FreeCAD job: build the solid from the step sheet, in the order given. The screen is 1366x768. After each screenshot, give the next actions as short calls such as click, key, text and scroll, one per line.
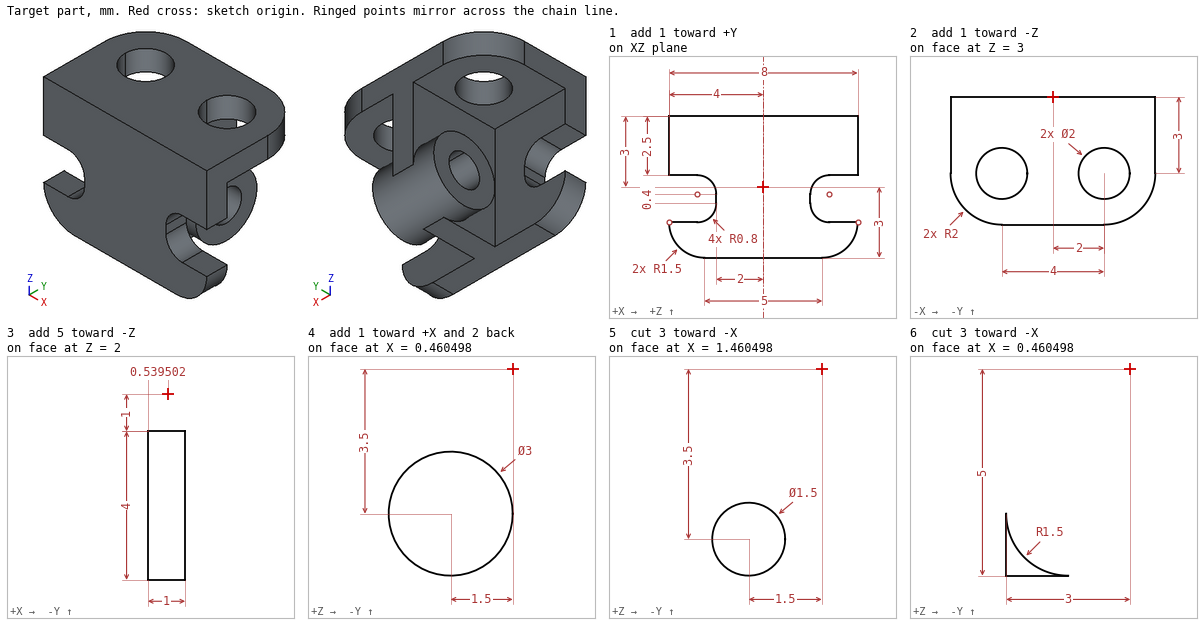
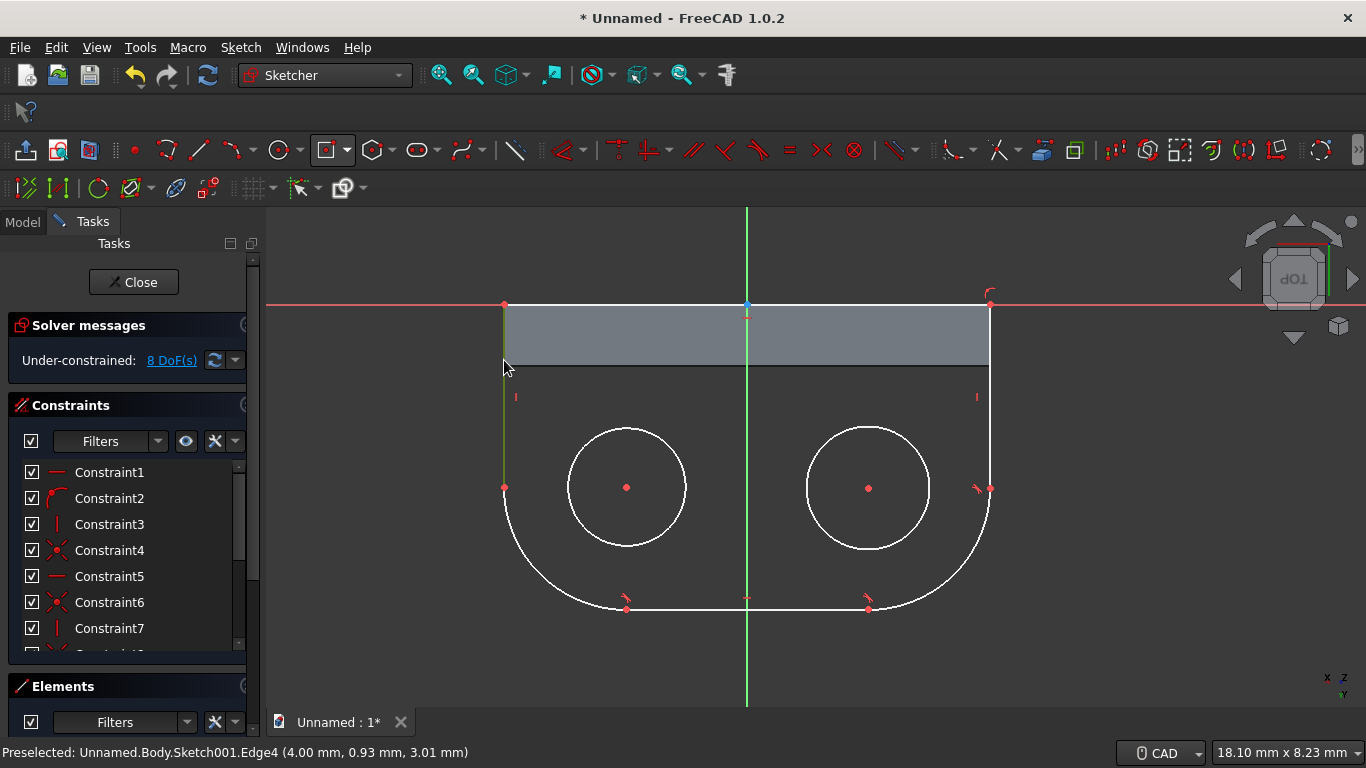
click(518, 543)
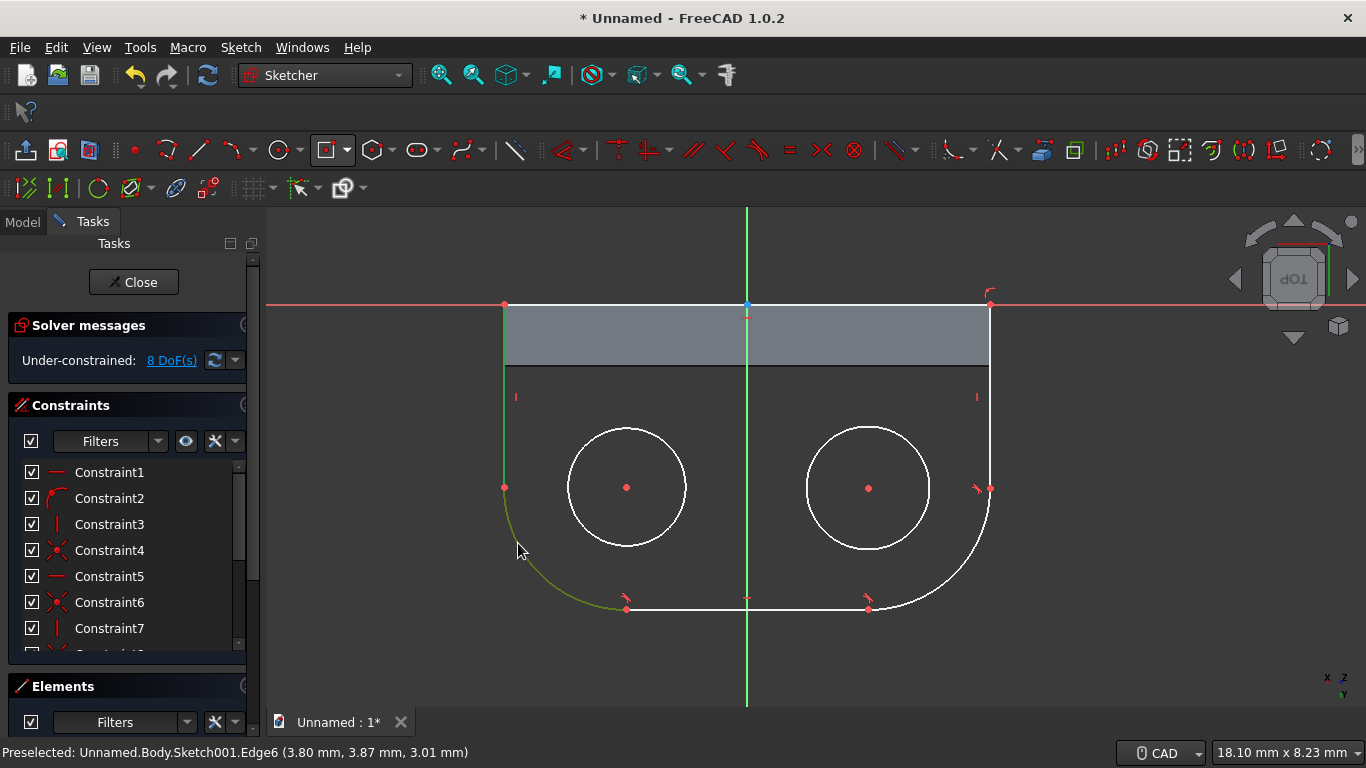
click(758, 150)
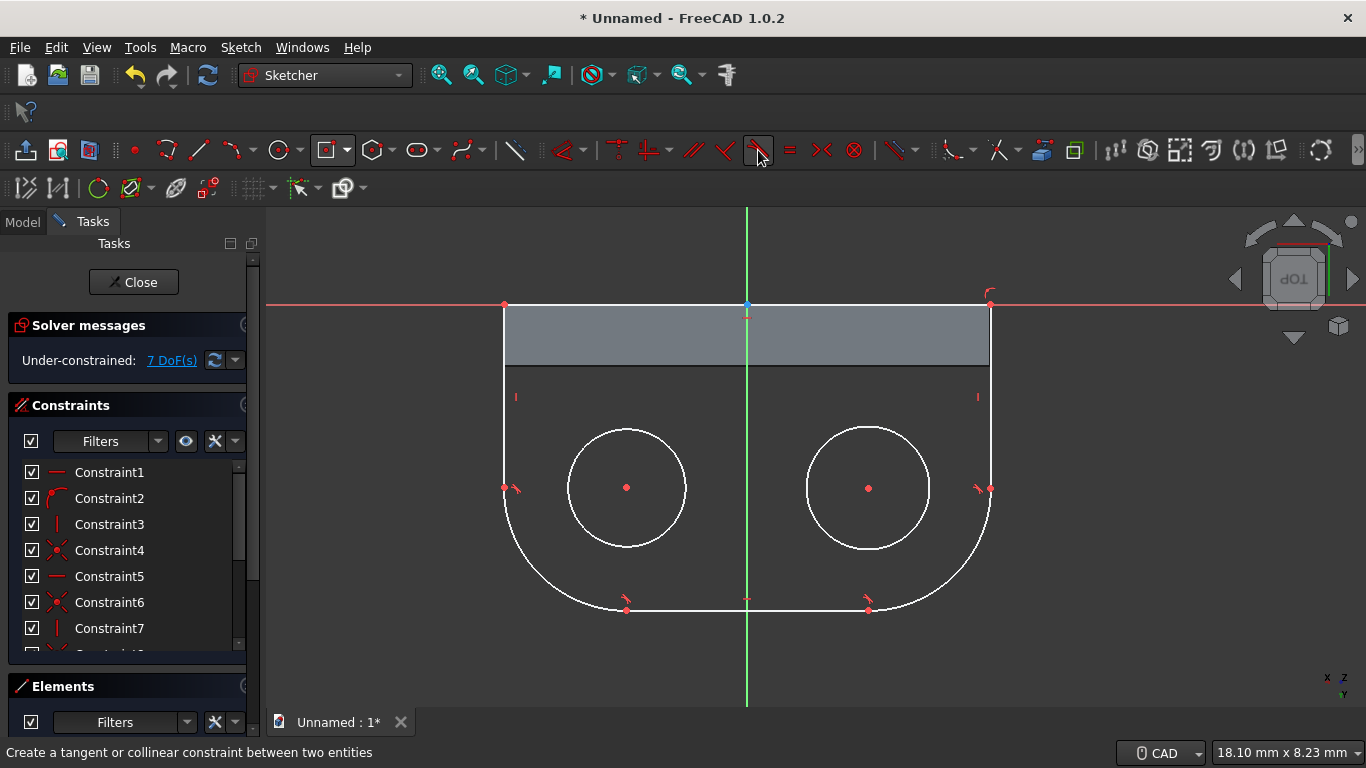
click(924, 598)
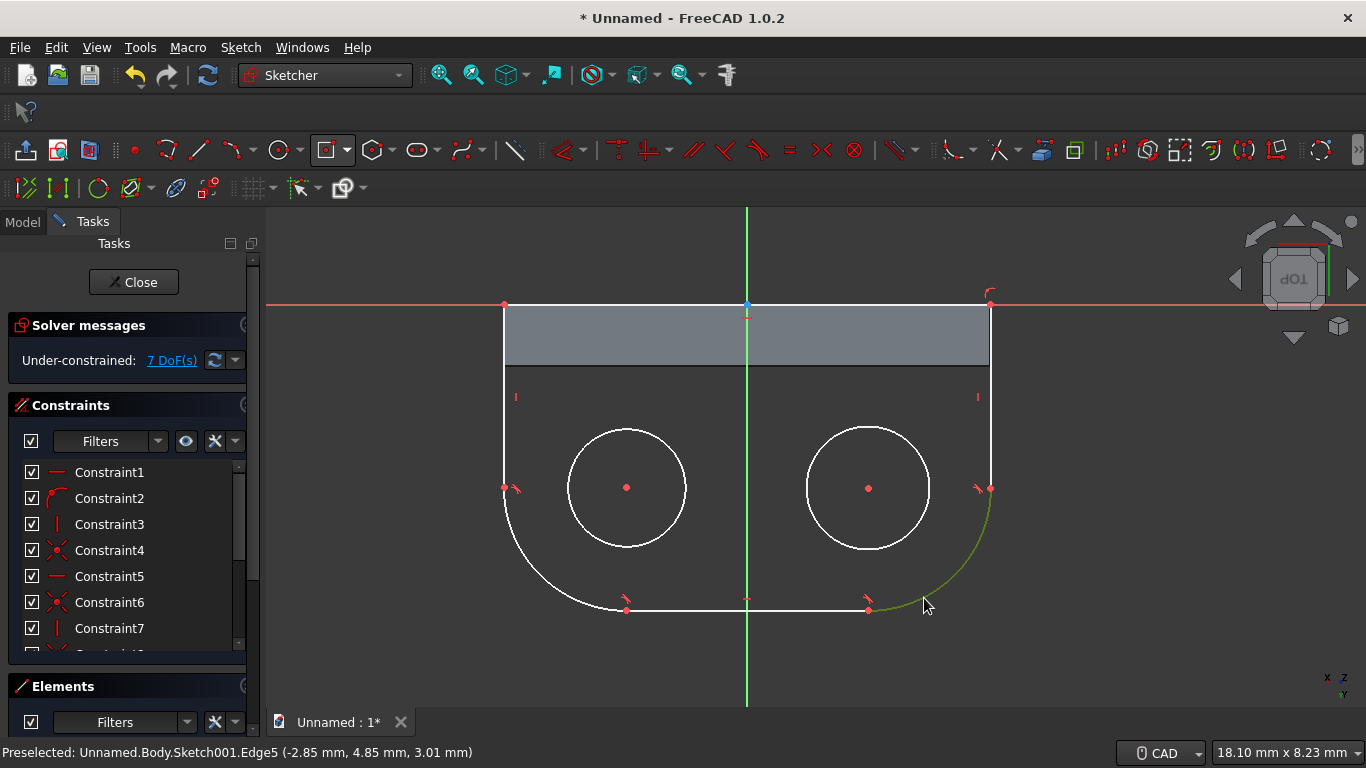
click(517, 544)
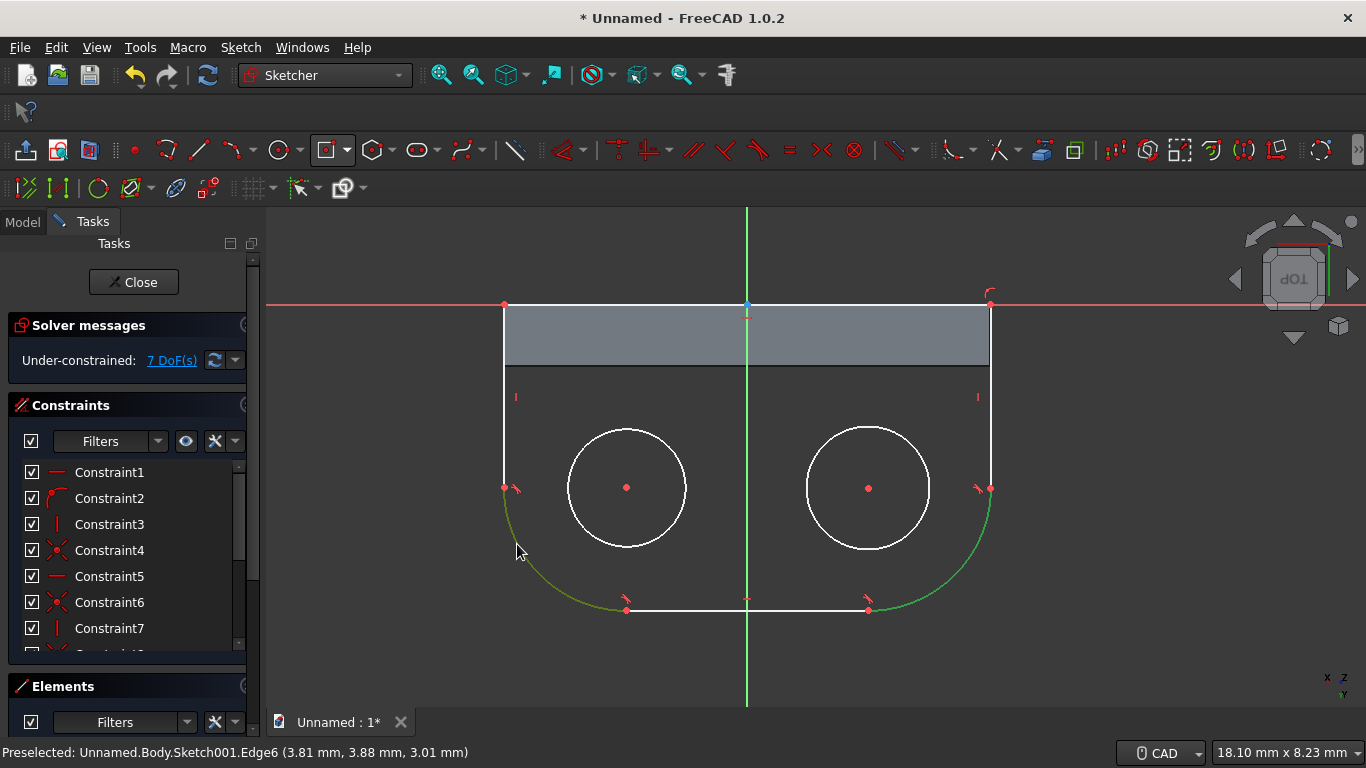
click(790, 150)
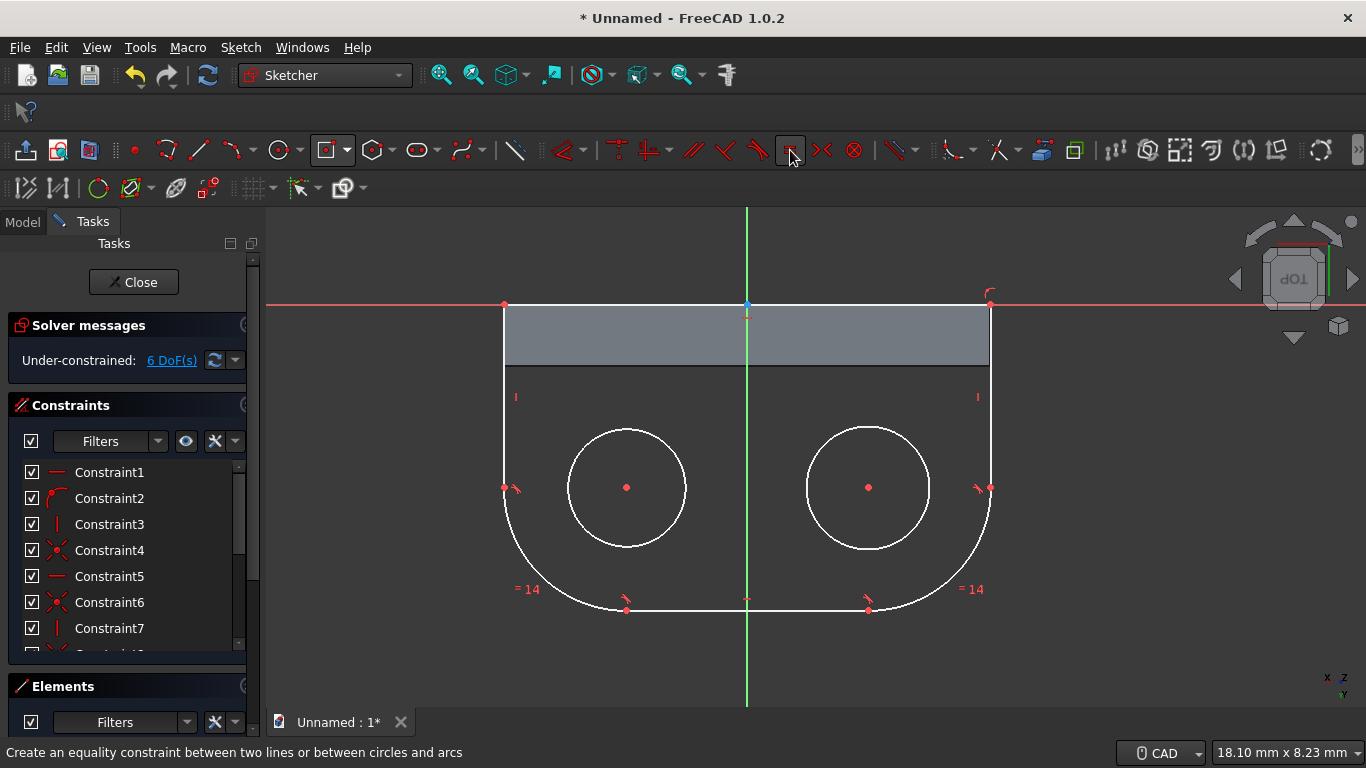
click(911, 444)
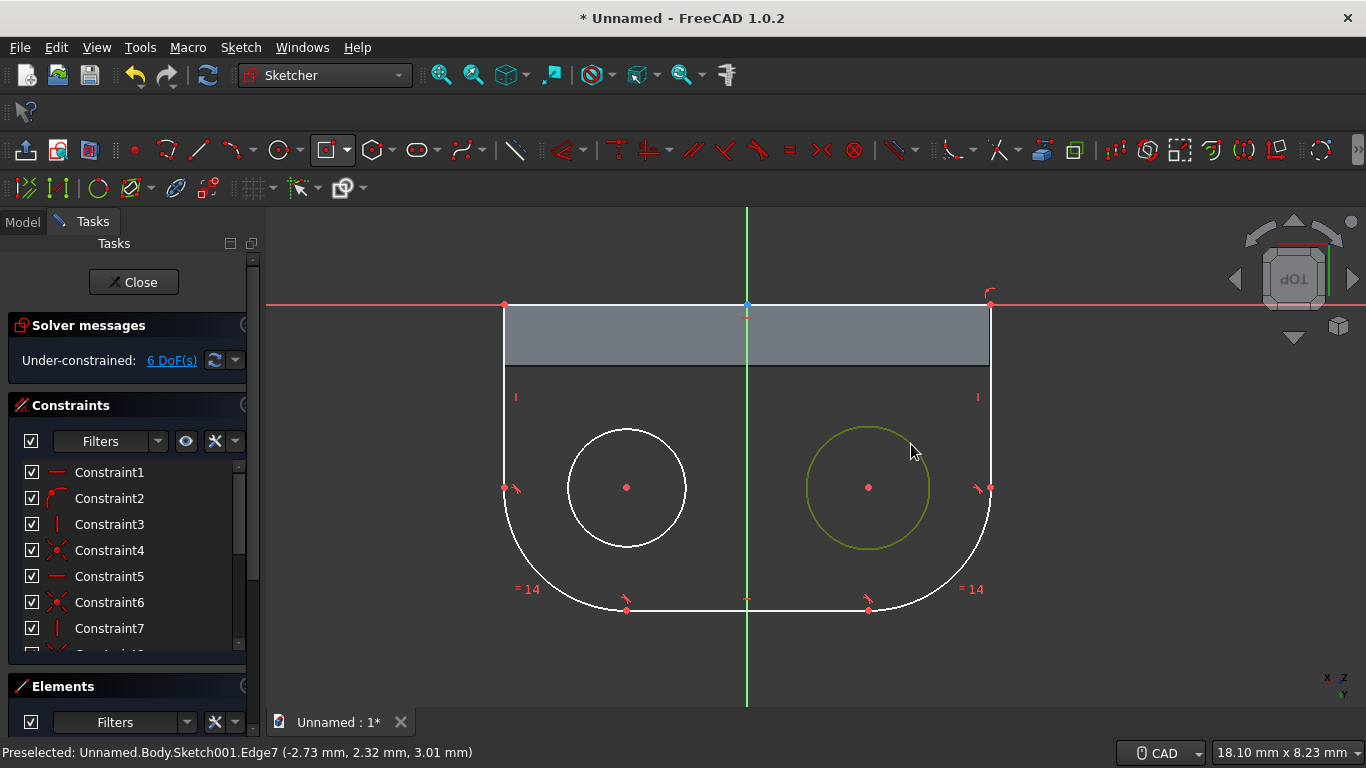
click(668, 446)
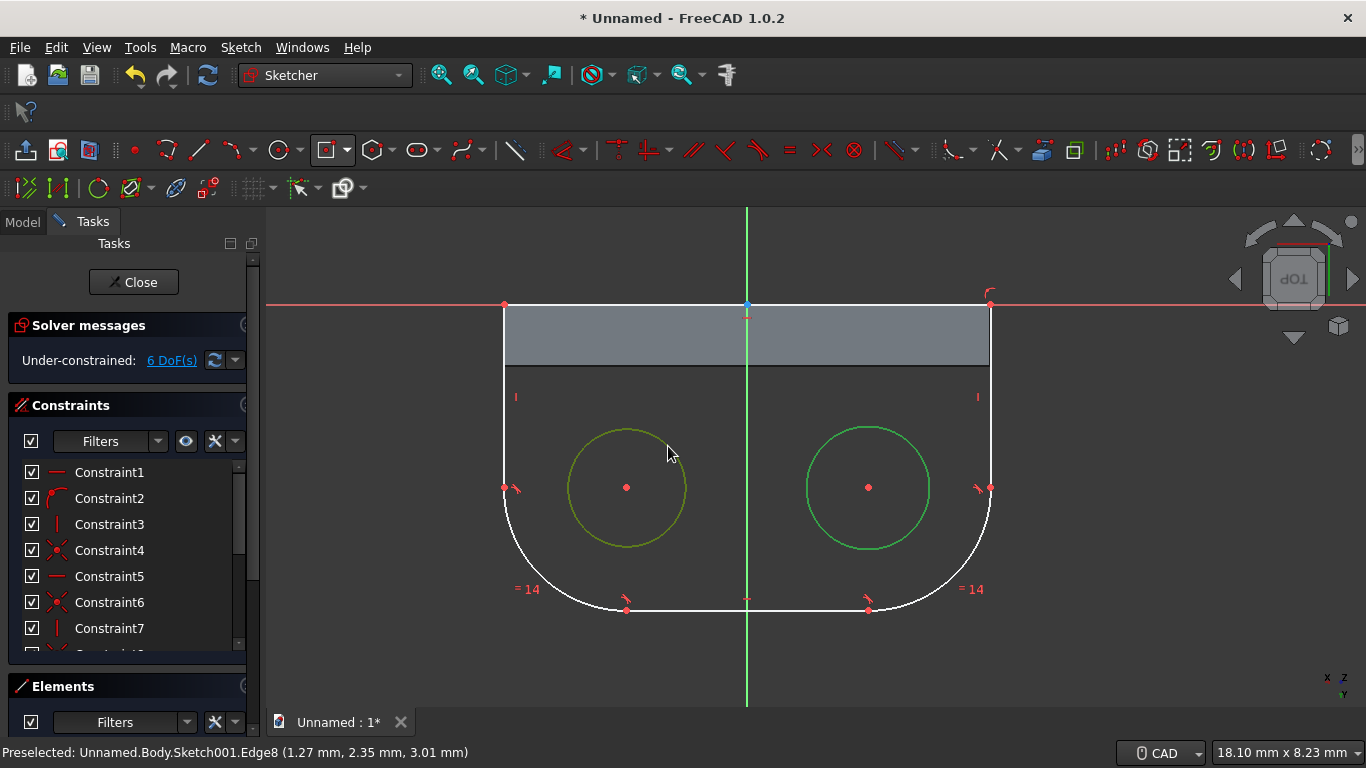
click(790, 150)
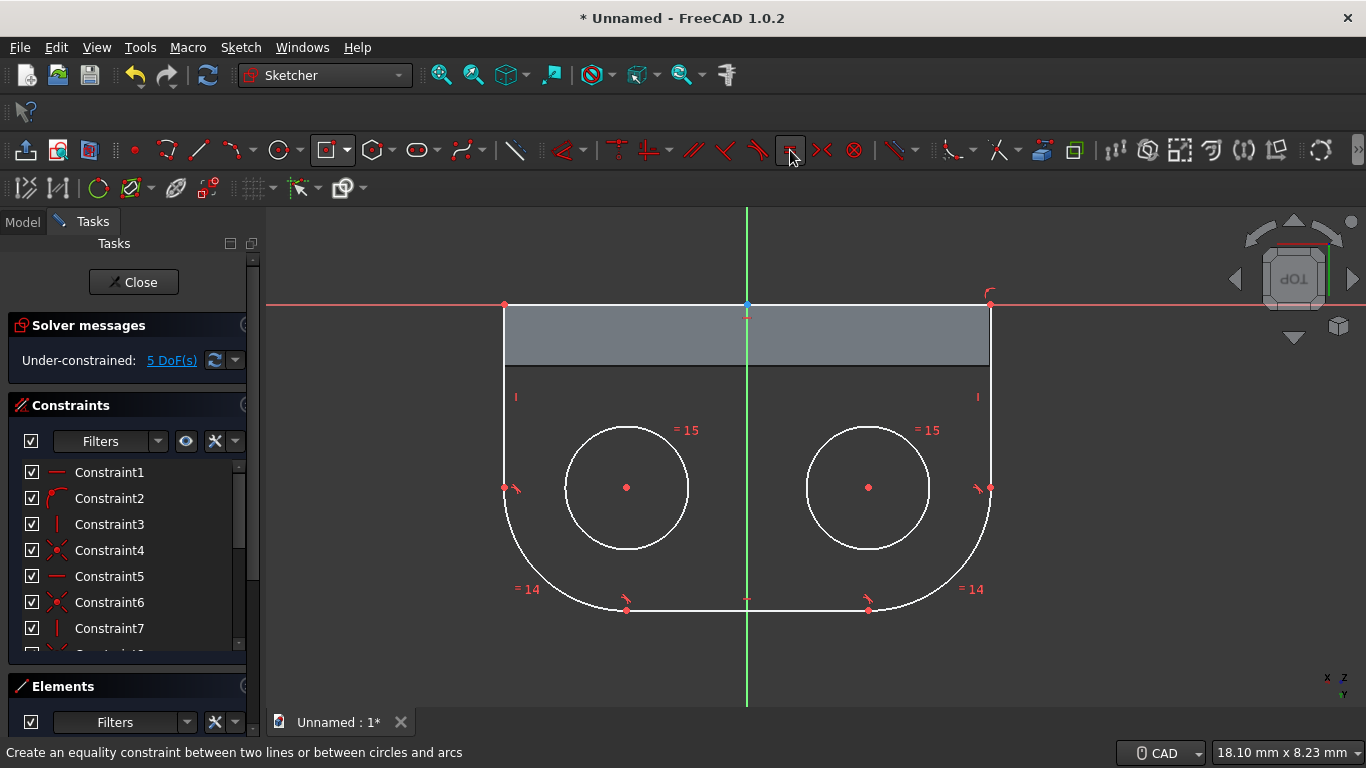
click(562, 150)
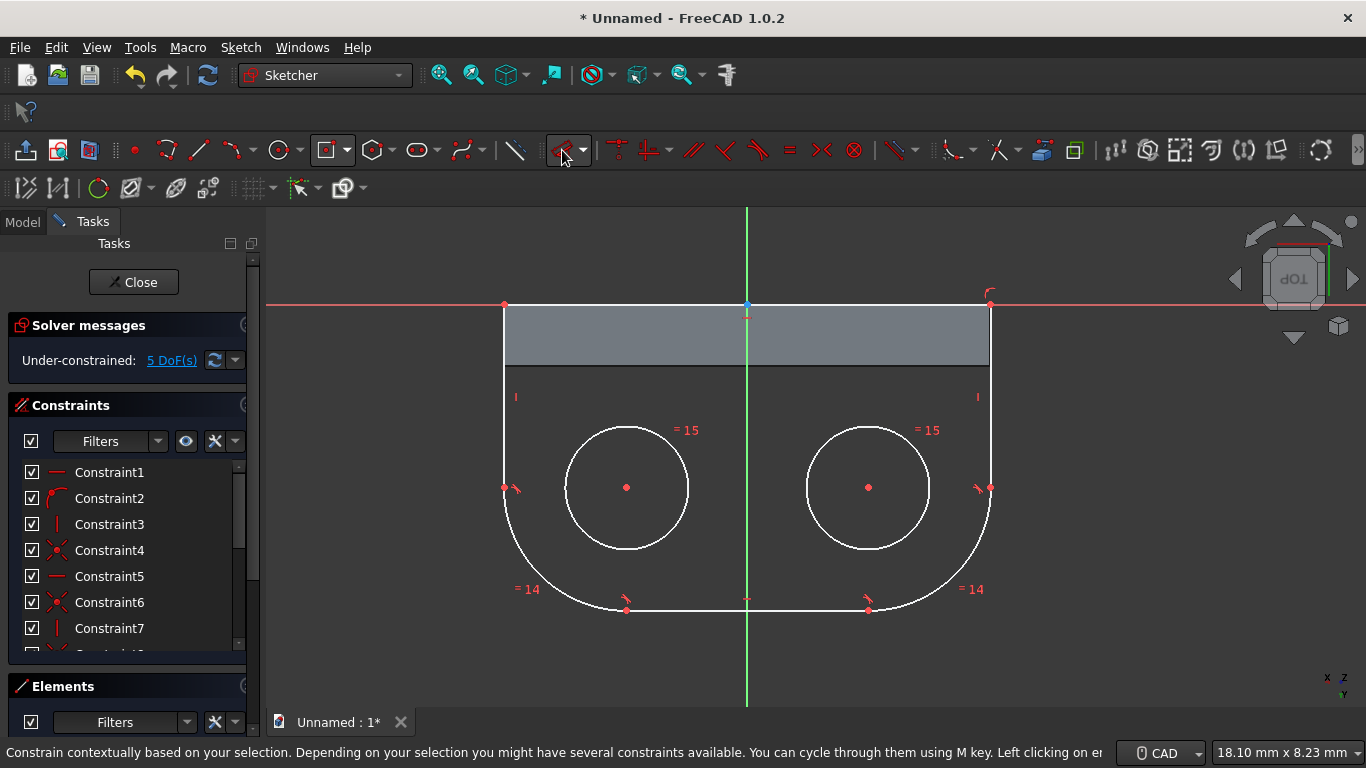
click(924, 598)
click(939, 627)